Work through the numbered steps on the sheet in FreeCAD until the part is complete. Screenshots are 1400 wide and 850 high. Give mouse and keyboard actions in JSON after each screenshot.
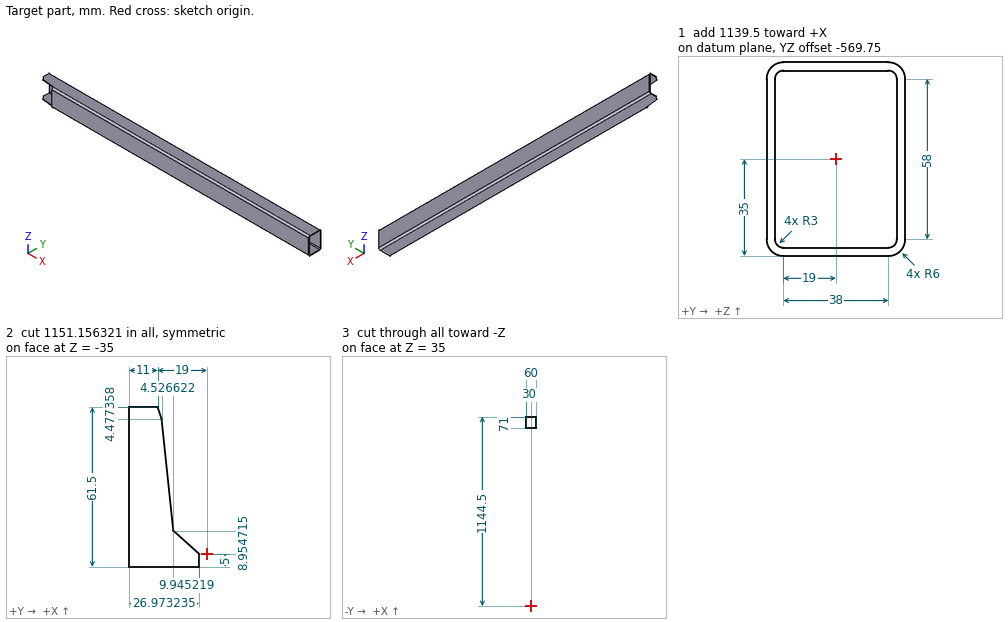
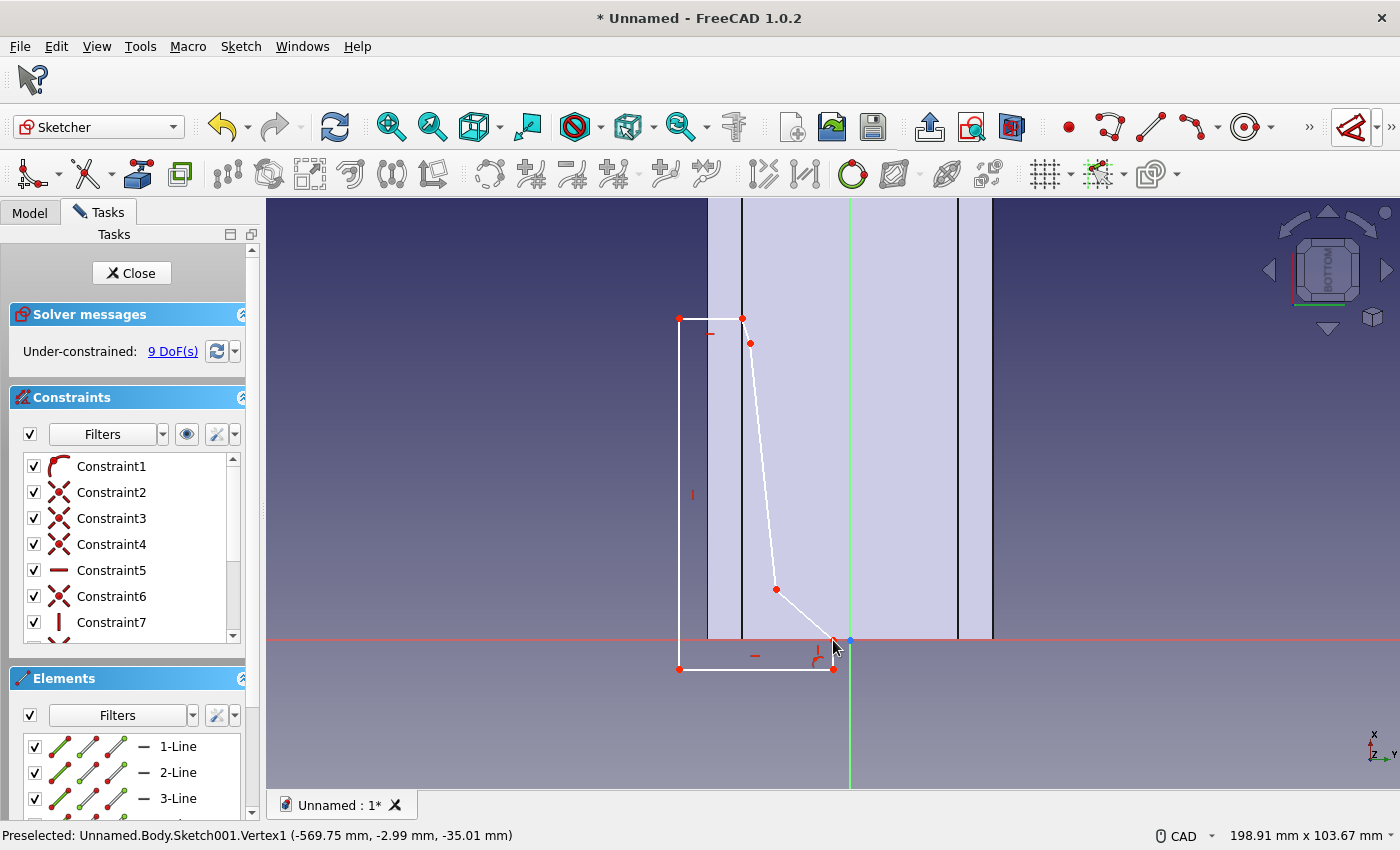
{"action": "scroll", "coordinate": [833, 658], "scroll_direction": "up", "scroll_amount": 2}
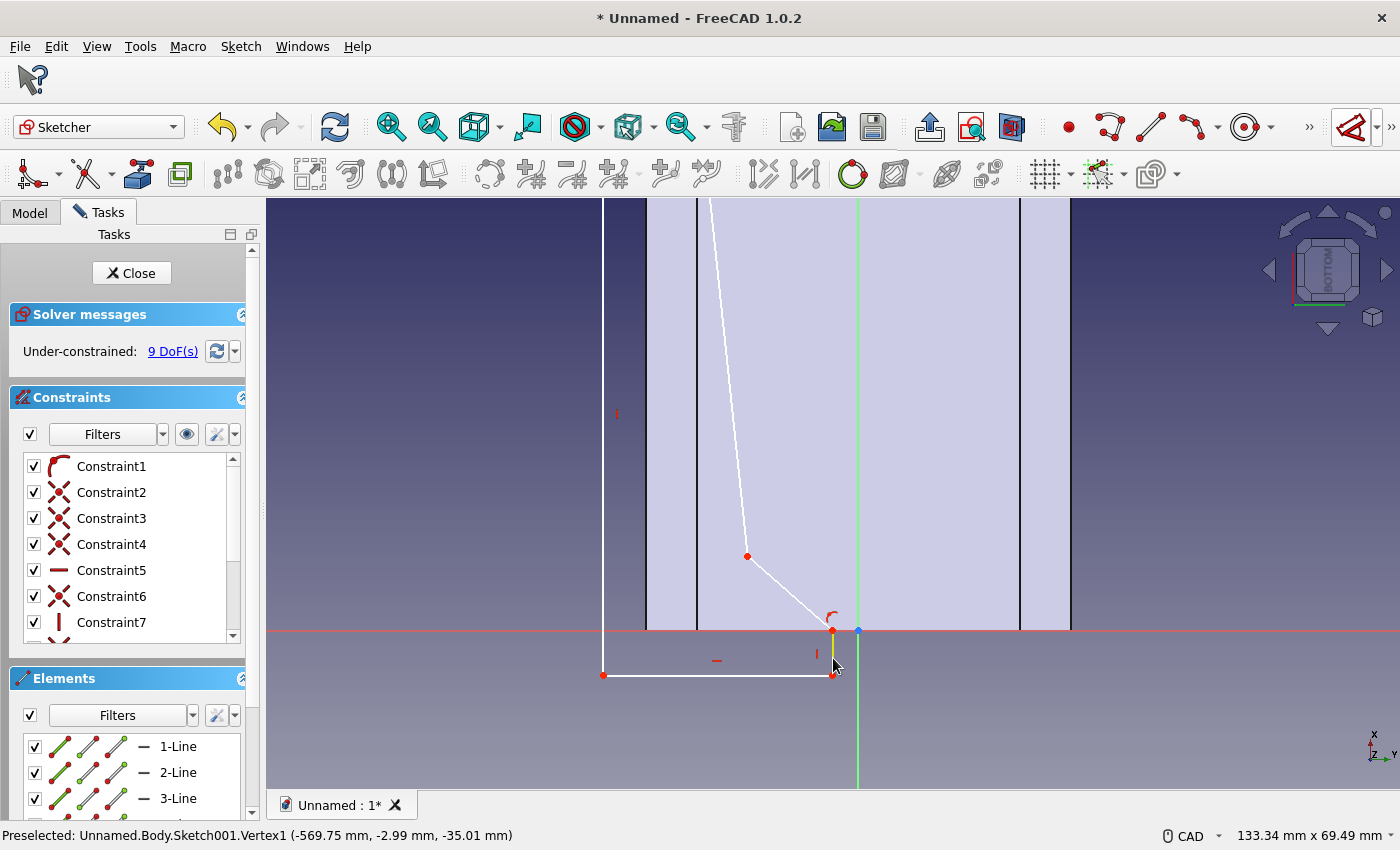
{"action": "left_click", "coordinate": [833, 658]}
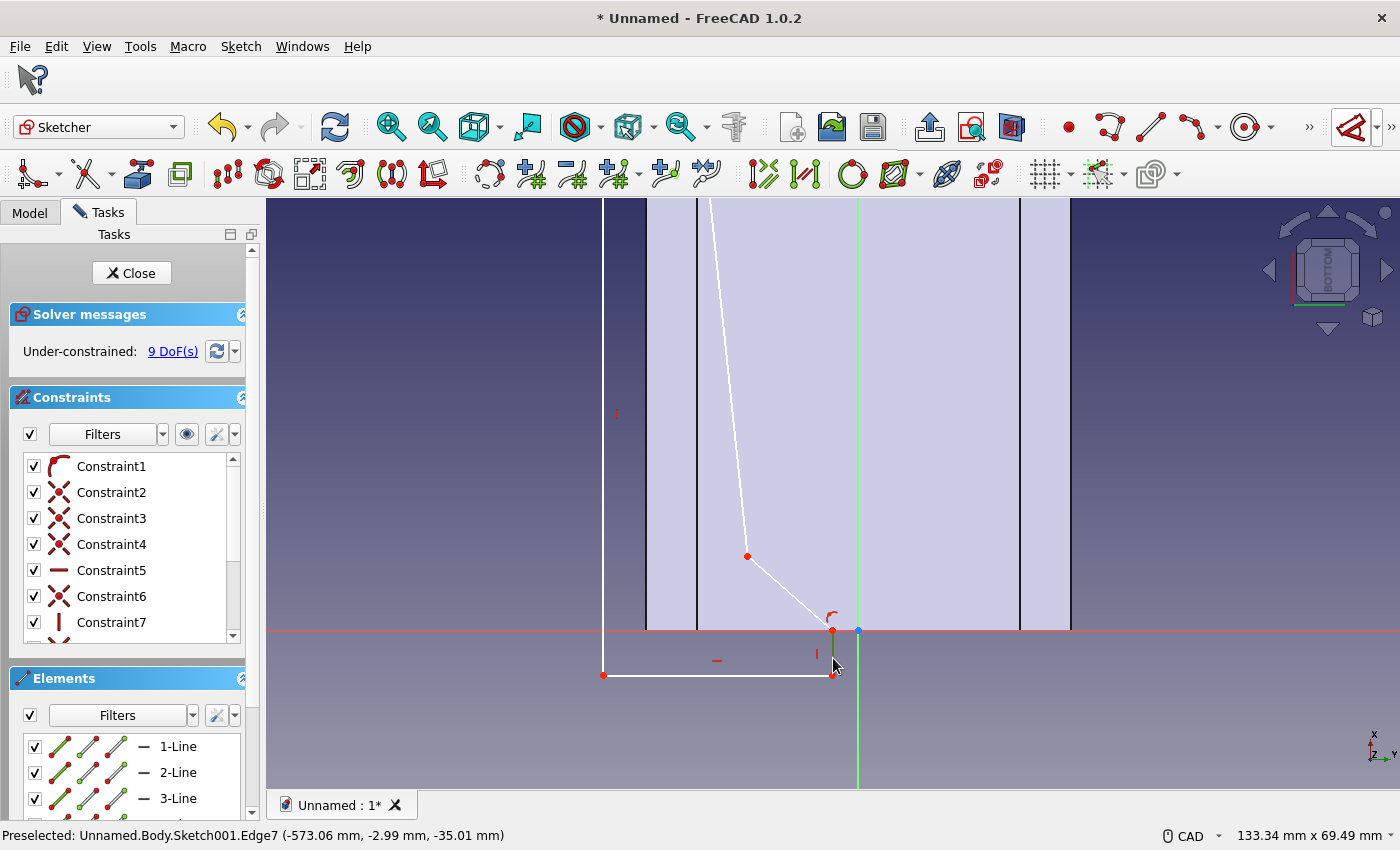
{"action": "key", "text": "i"}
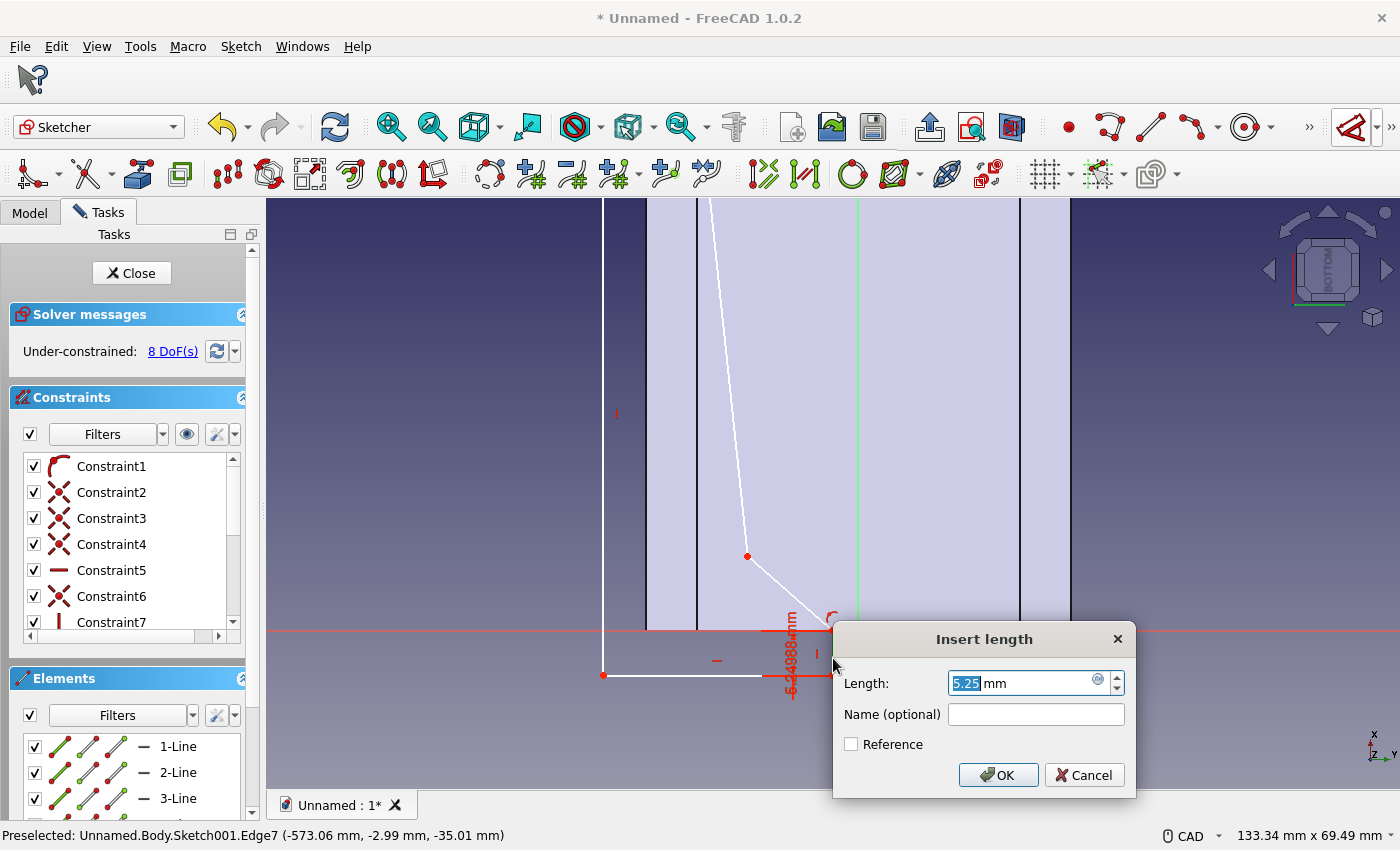
{"action": "type", "text": "5"}
{"action": "key", "text": "Return"}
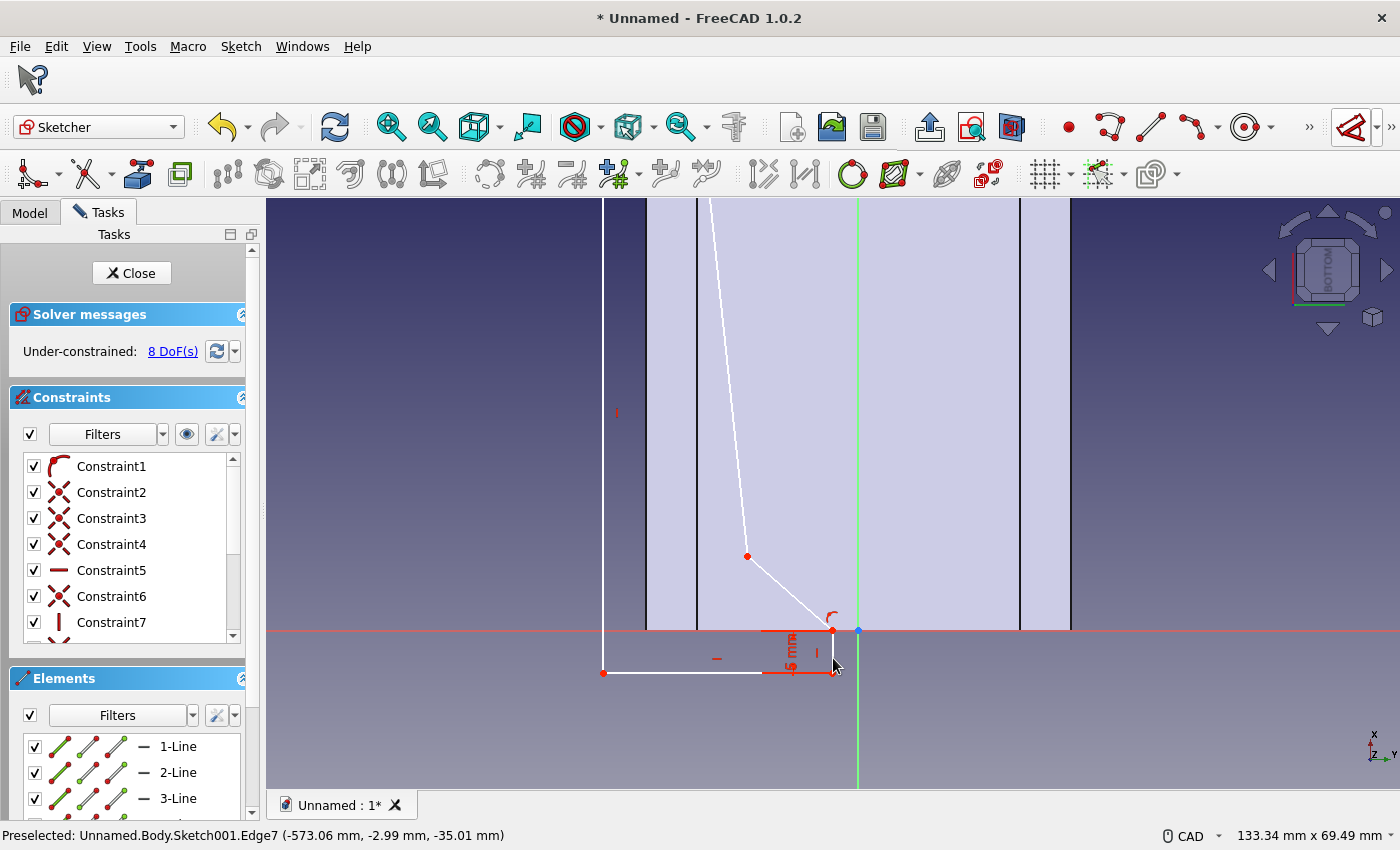
{"action": "scroll", "coordinate": [833, 659], "scroll_direction": "down", "scroll_amount": 2}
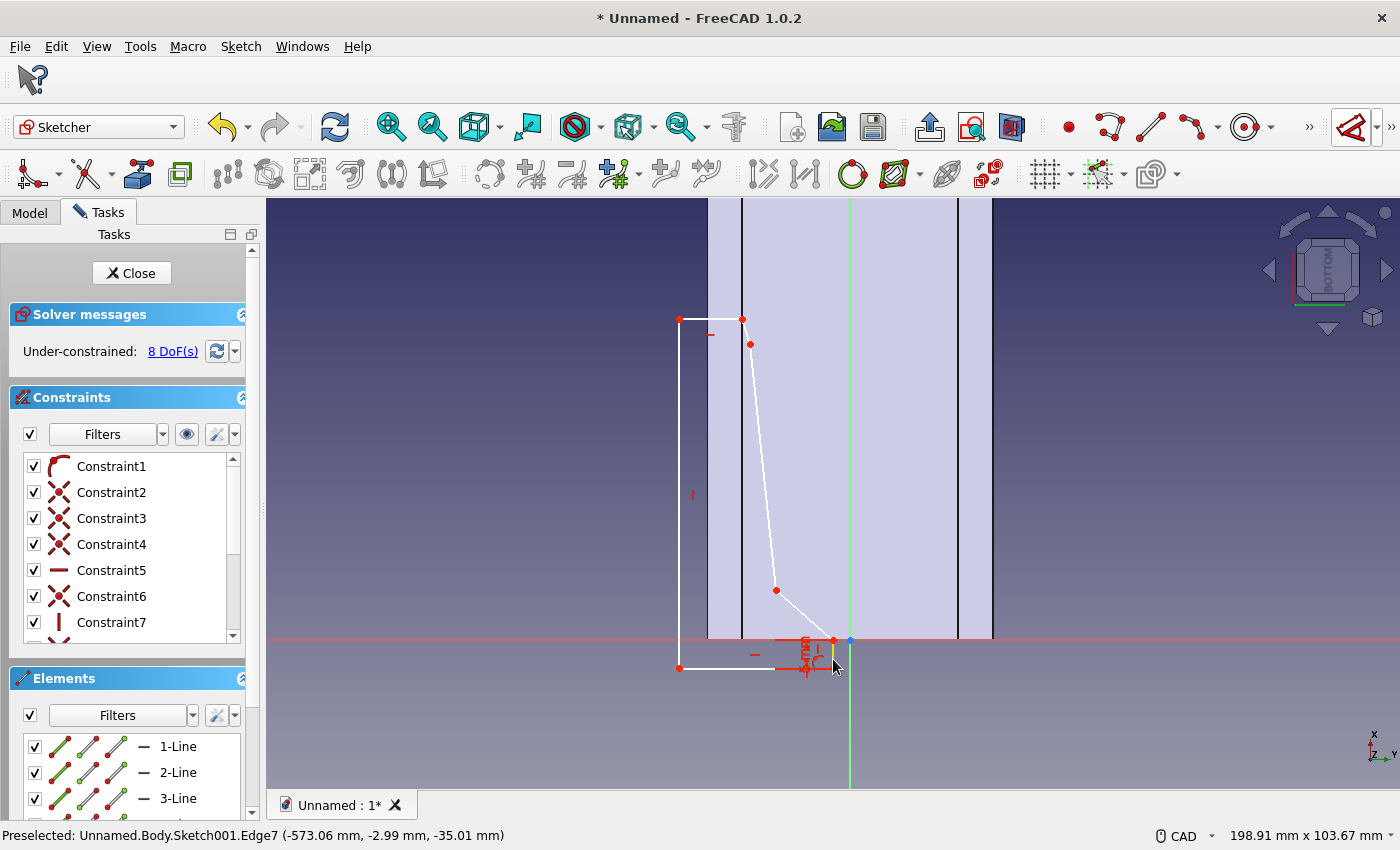
{"action": "left_click", "coordinate": [723, 319]}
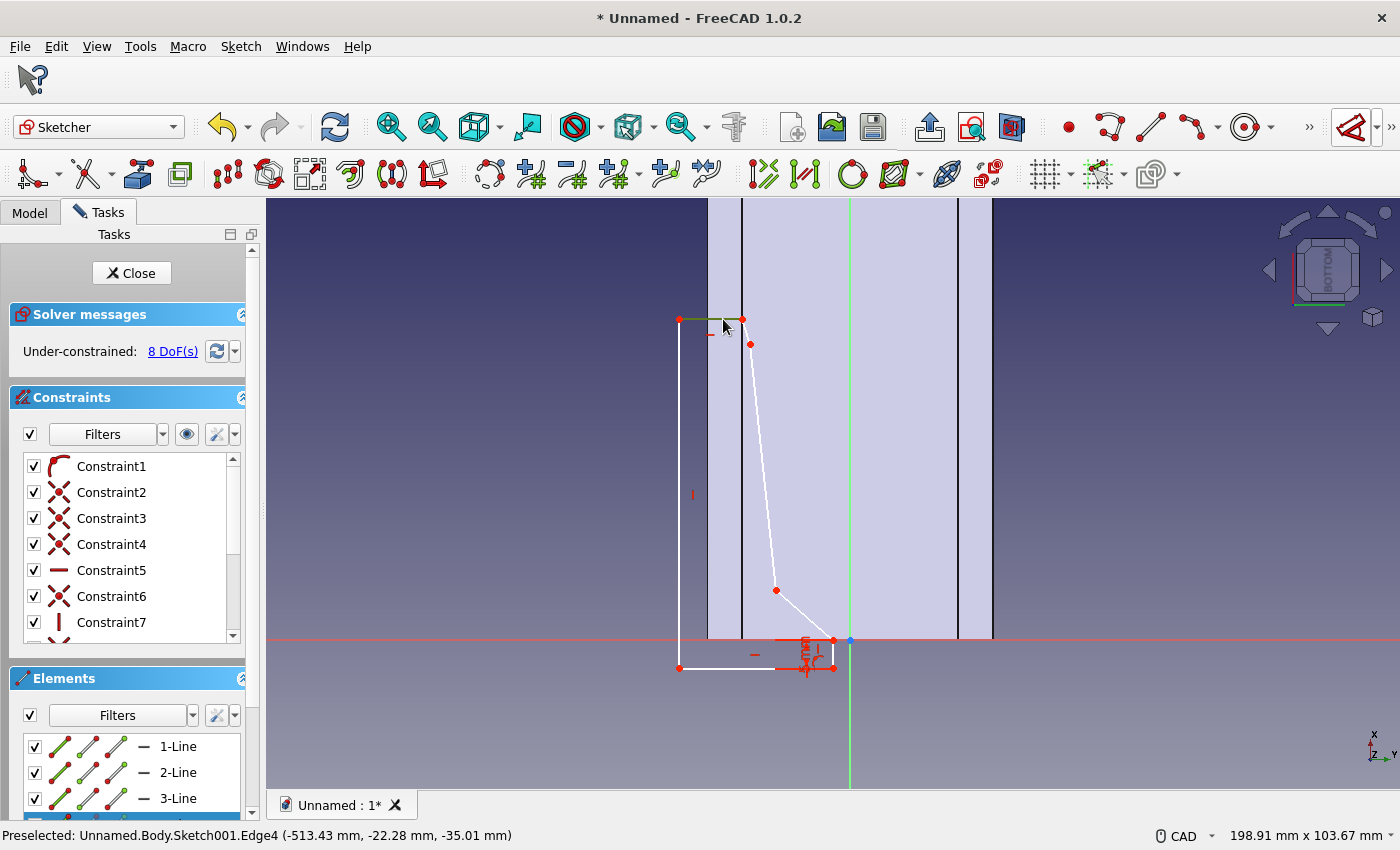
{"action": "key", "text": "l"}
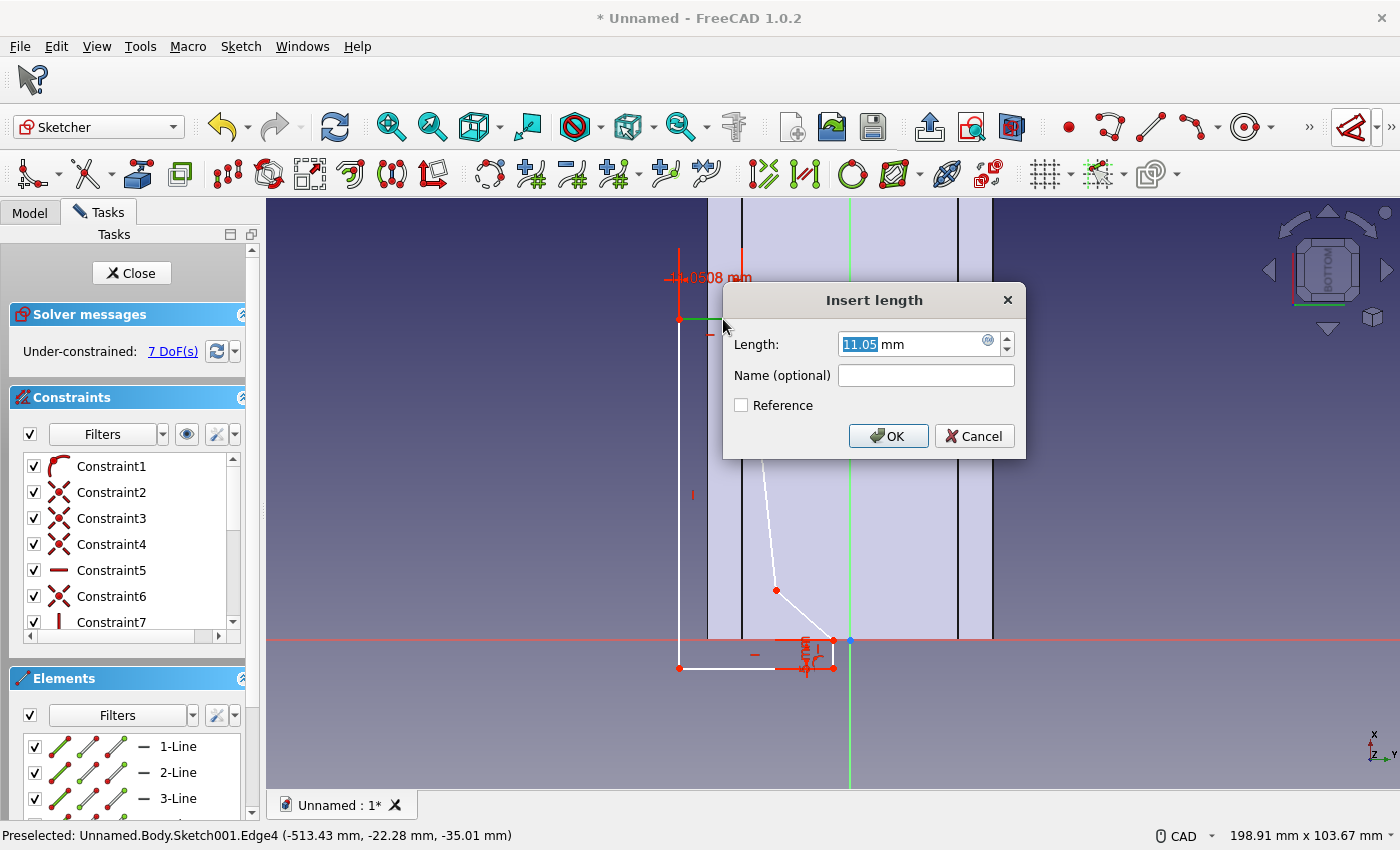
{"action": "type", "text": "11"}
{"action": "key", "text": "Return"}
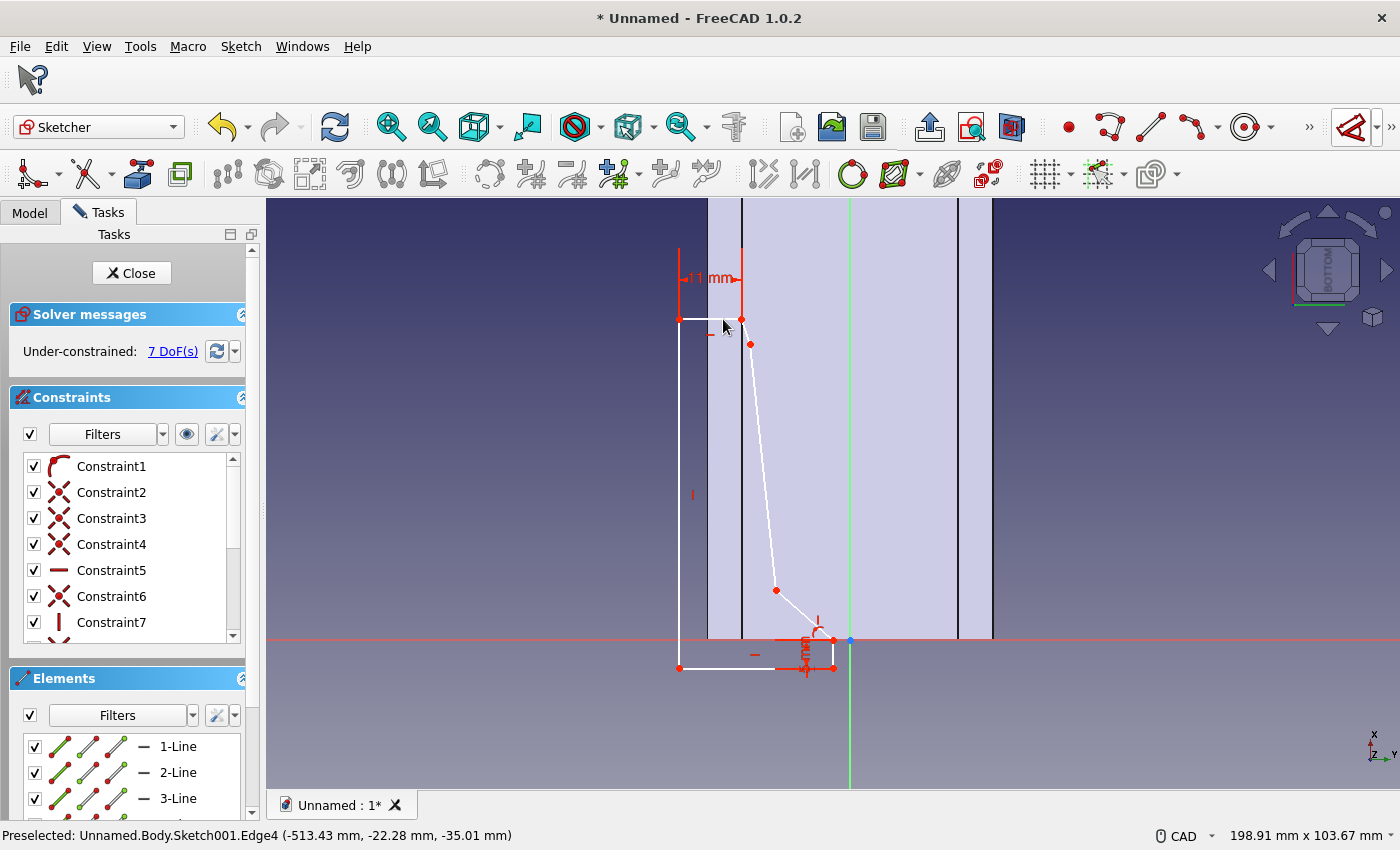
{"action": "left_click", "coordinate": [742, 319]}